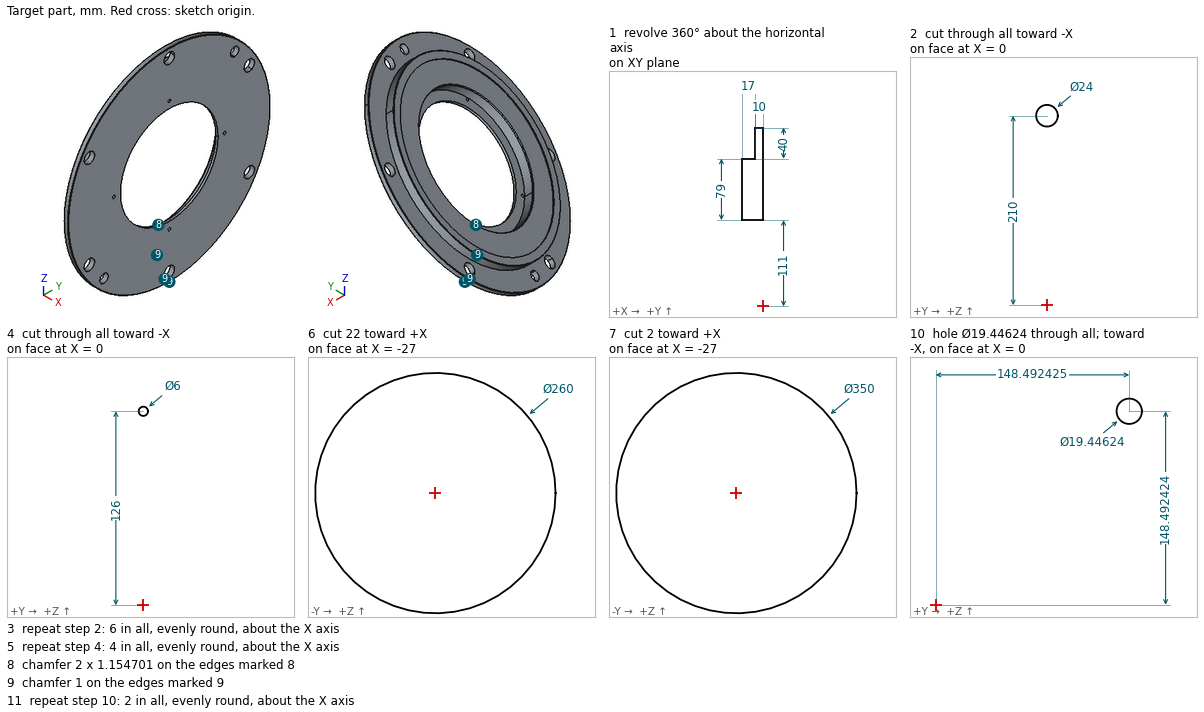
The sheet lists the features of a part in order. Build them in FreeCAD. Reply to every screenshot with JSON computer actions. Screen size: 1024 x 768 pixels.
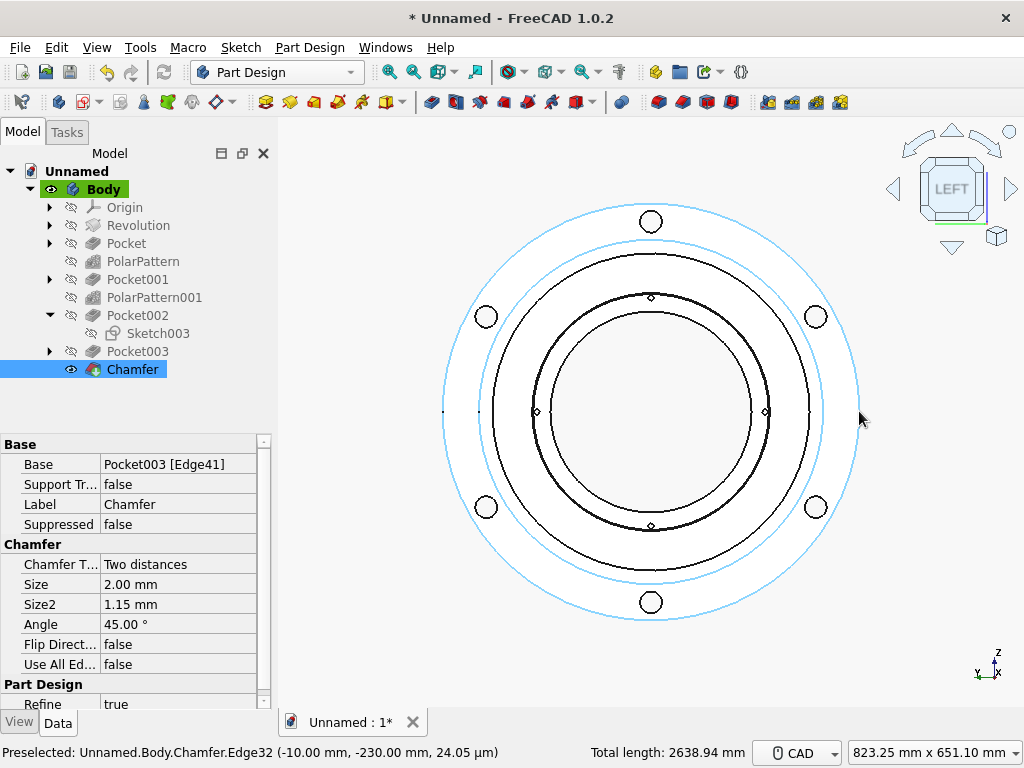
{"action": "key", "text": "0"}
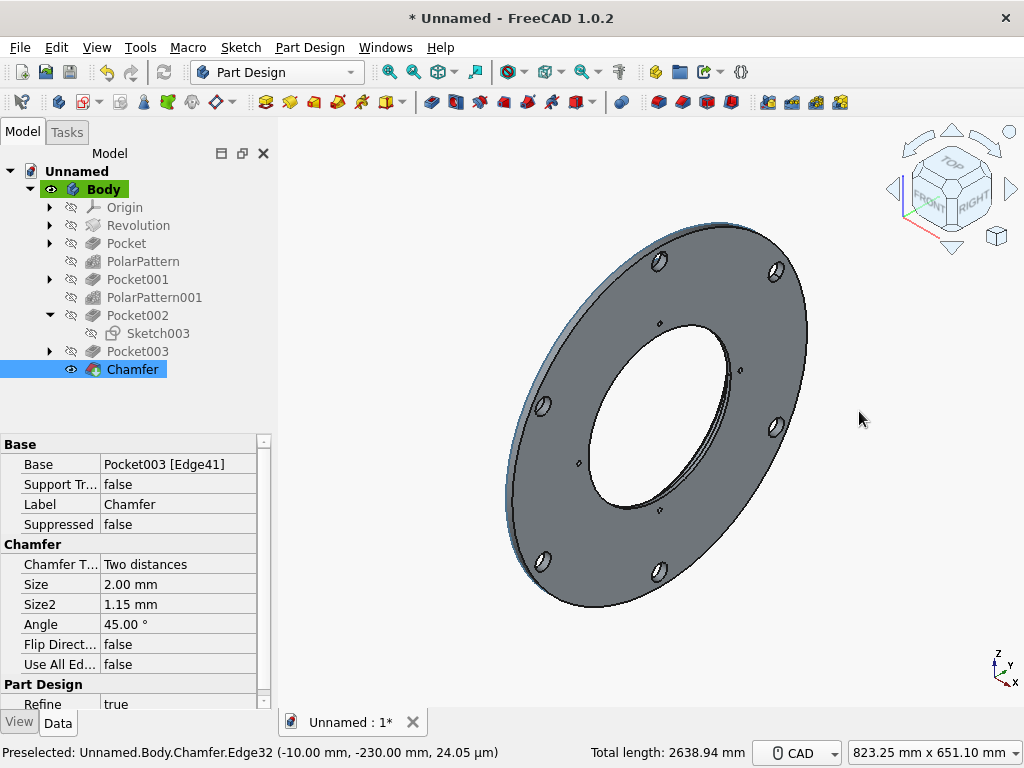
{"action": "left_click", "coordinate": [512, 501], "text": "ctrl"}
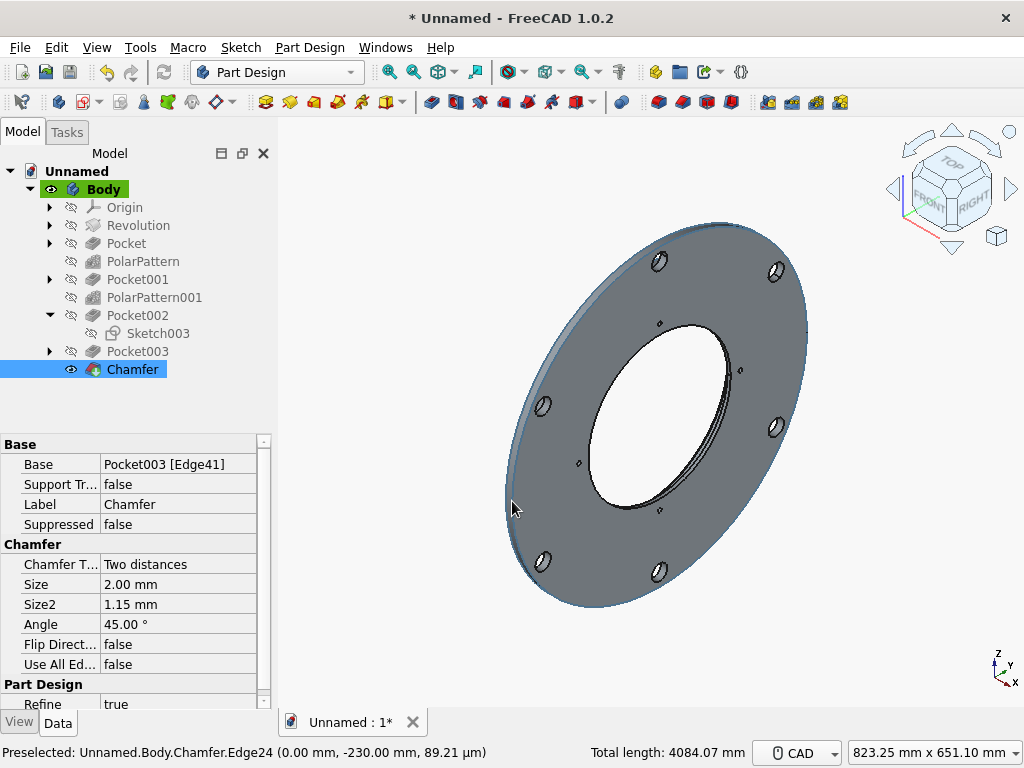
{"action": "left_click", "coordinate": [684, 102]}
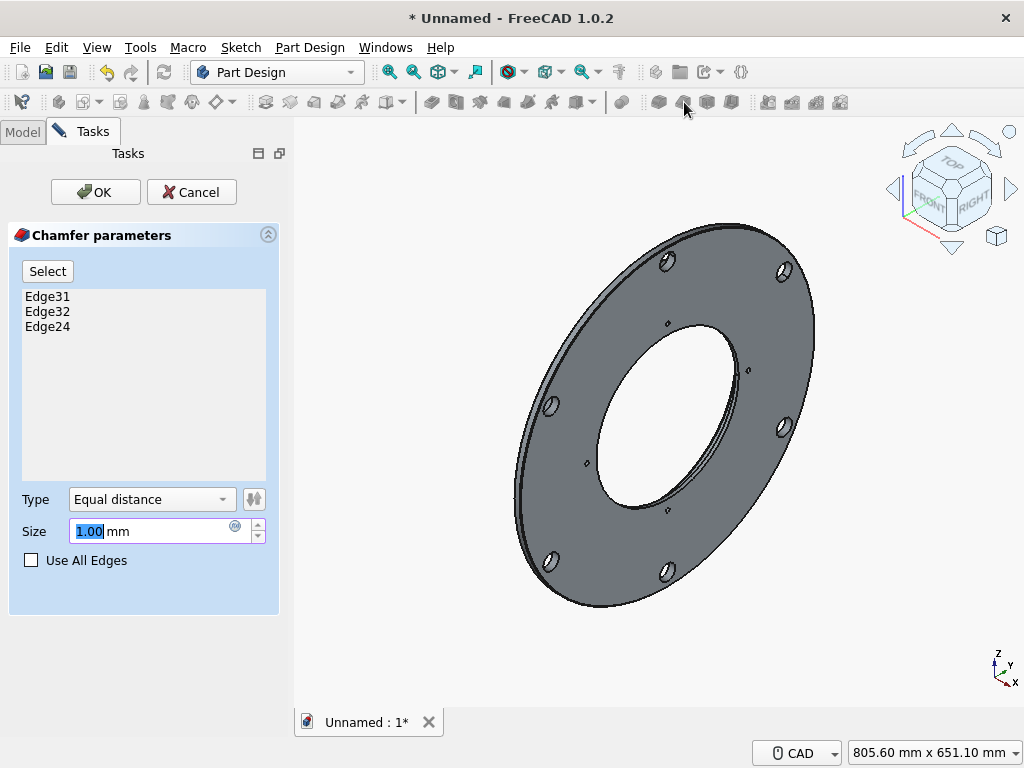
{"action": "type", "text": "1"}
{"action": "key", "text": "Tab"}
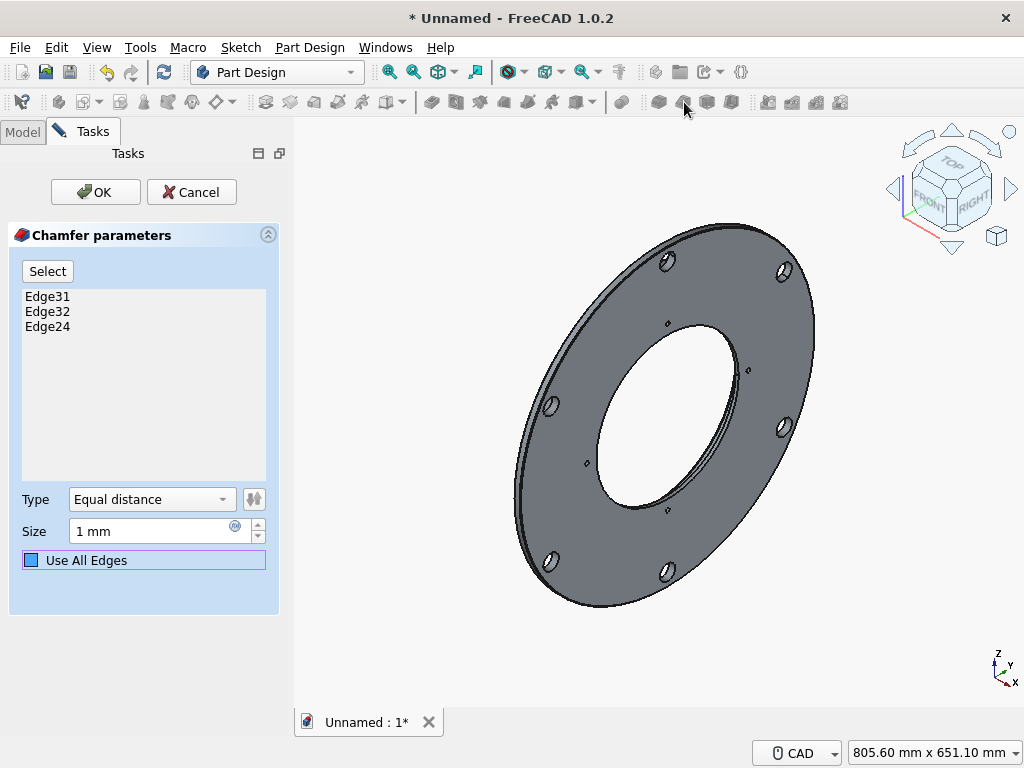
{"action": "left_click", "coordinate": [96, 192]}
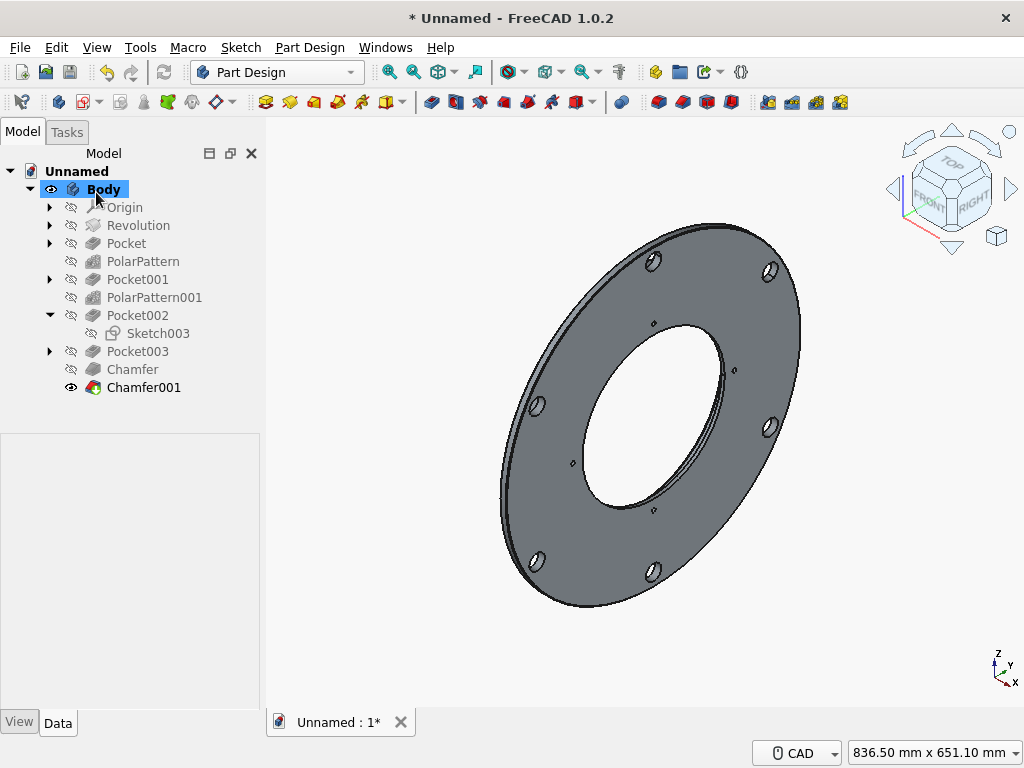
{"action": "left_click", "coordinate": [737, 271]}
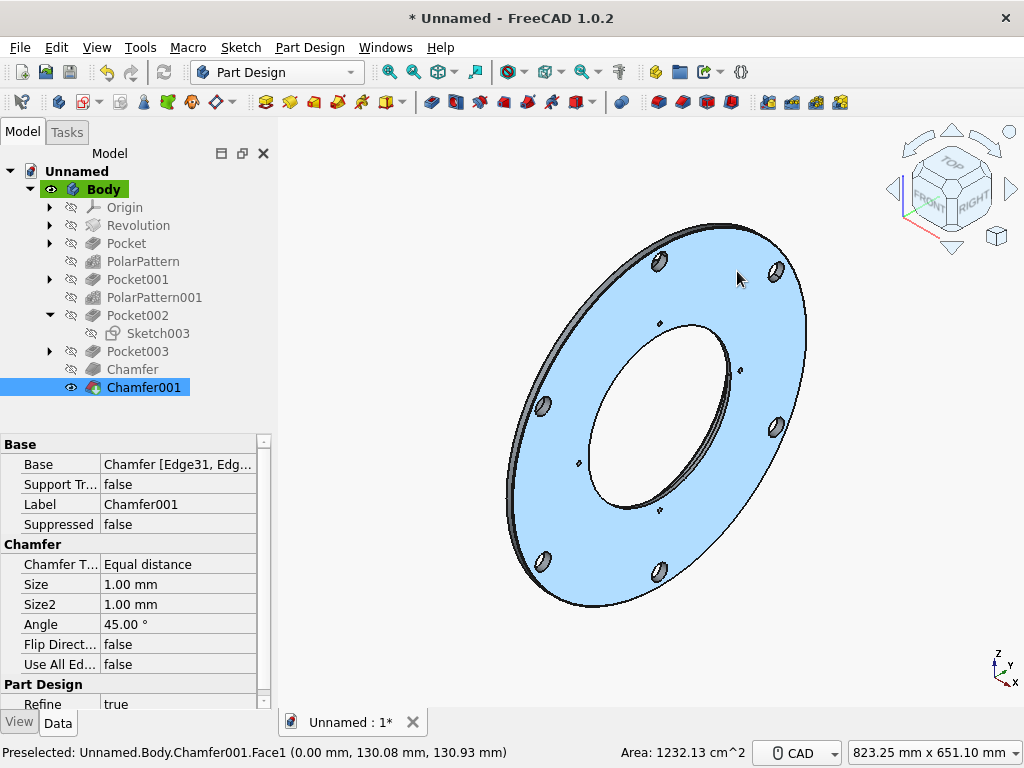
{"action": "left_click", "coordinate": [84, 102]}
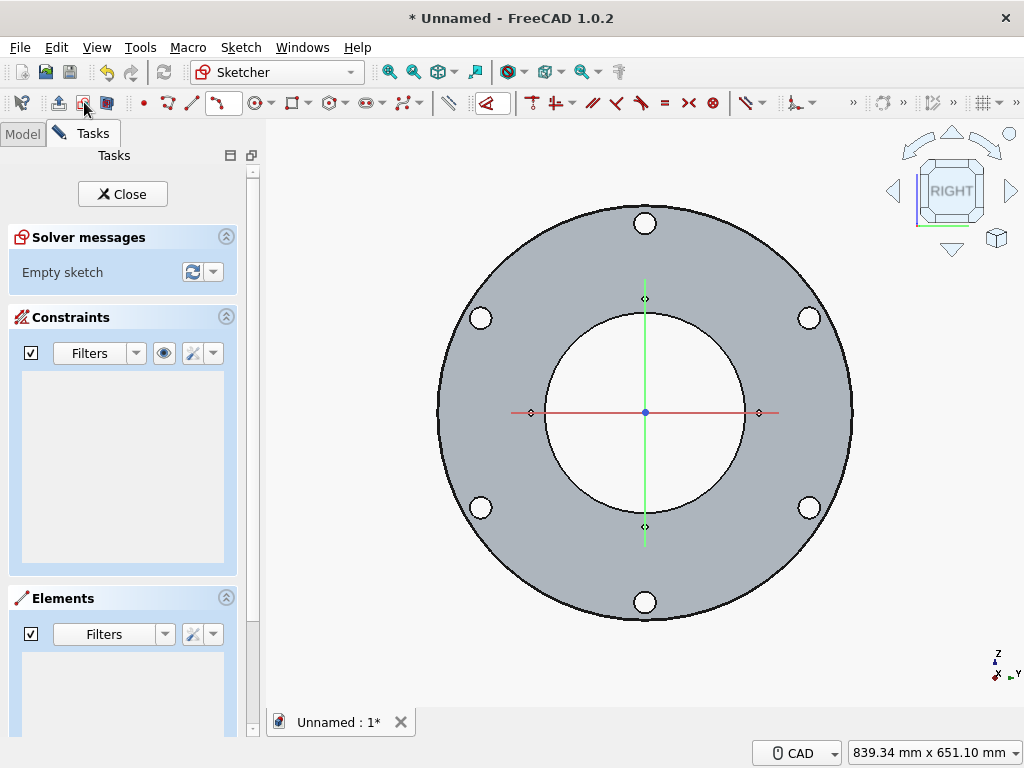
{"action": "scroll", "coordinate": [790, 272], "scroll_direction": "up", "scroll_amount": 15}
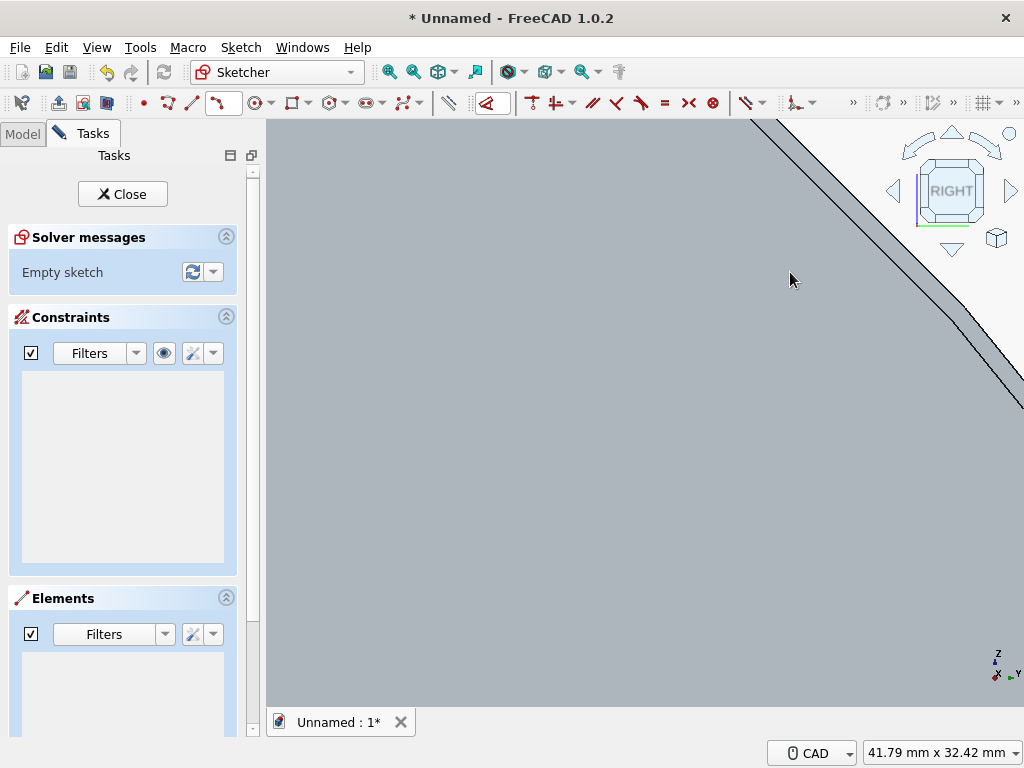
{"action": "left_click", "coordinate": [256, 104]}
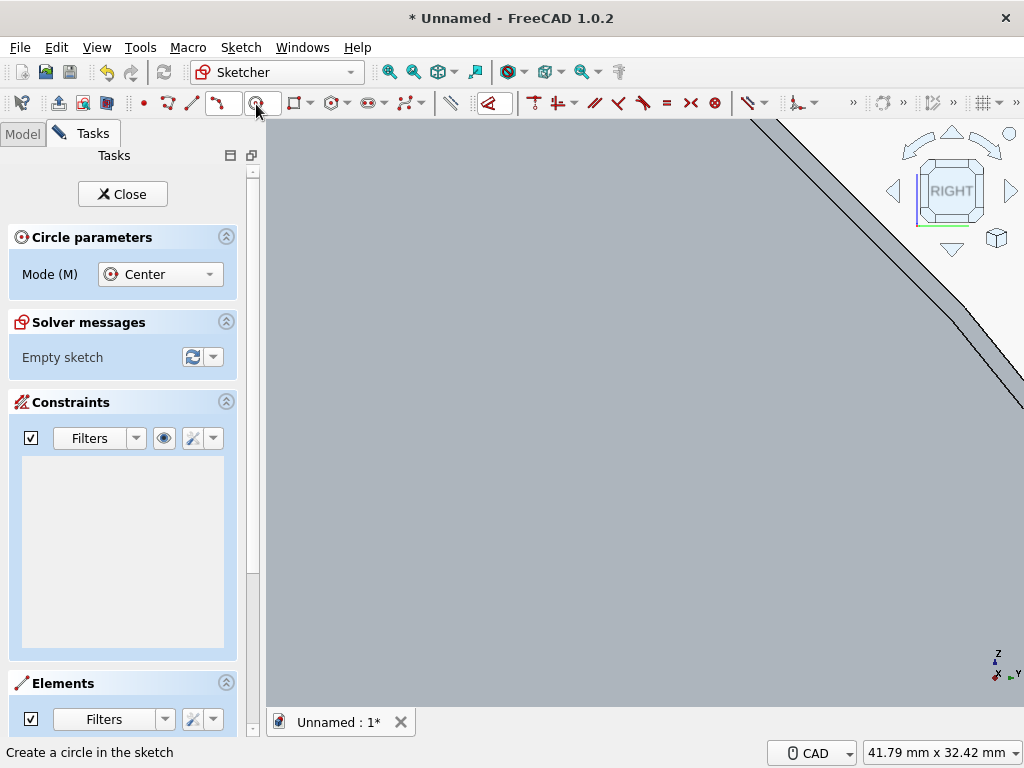
{"action": "left_click", "coordinate": [558, 406]}
{"action": "mouse_move", "coordinate": [683, 281]}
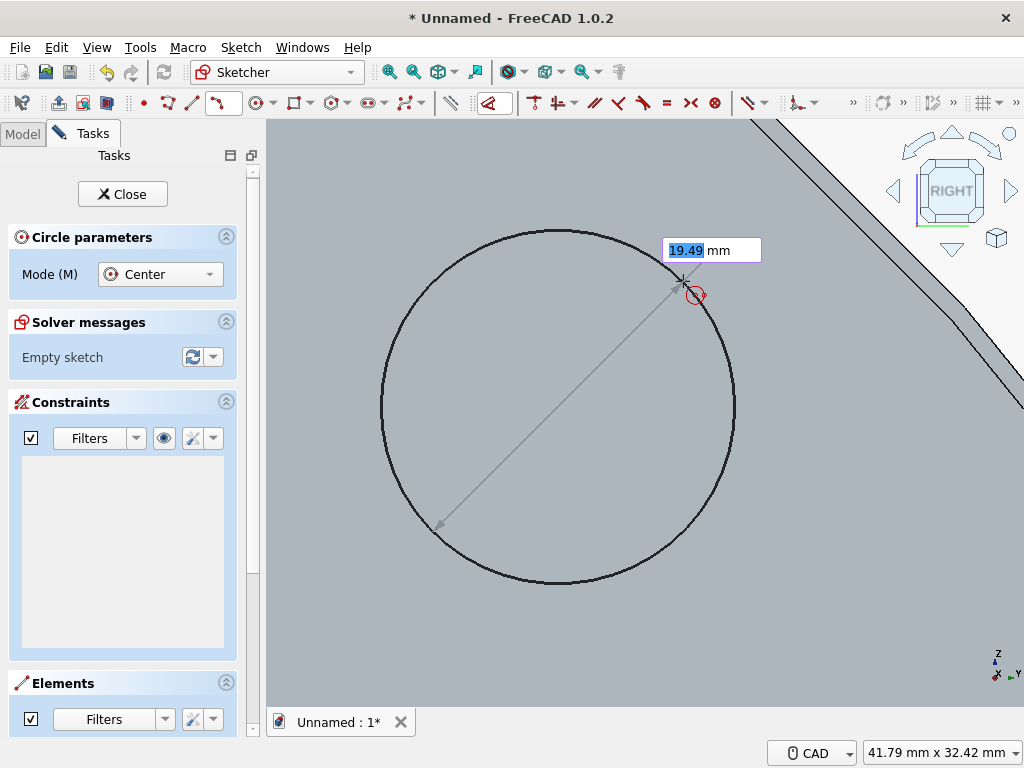
{"action": "type", "text": "19.44624"}
{"action": "key", "text": "Return"}
{"action": "key", "text": "Escape"}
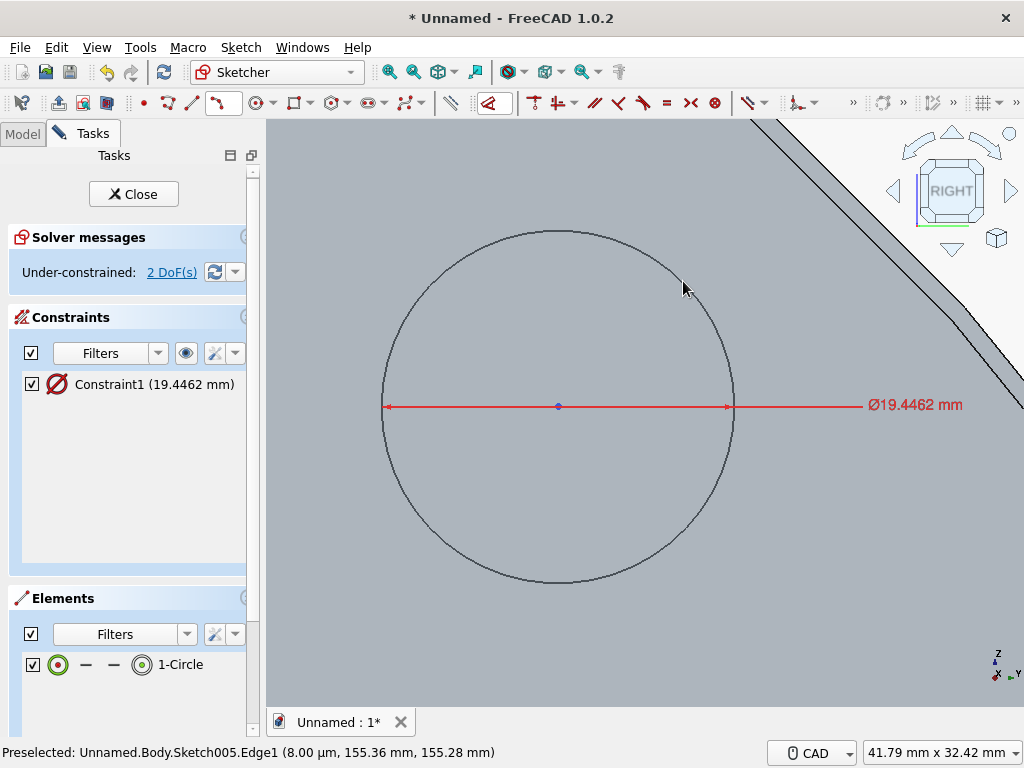
{"action": "key", "text": "d"}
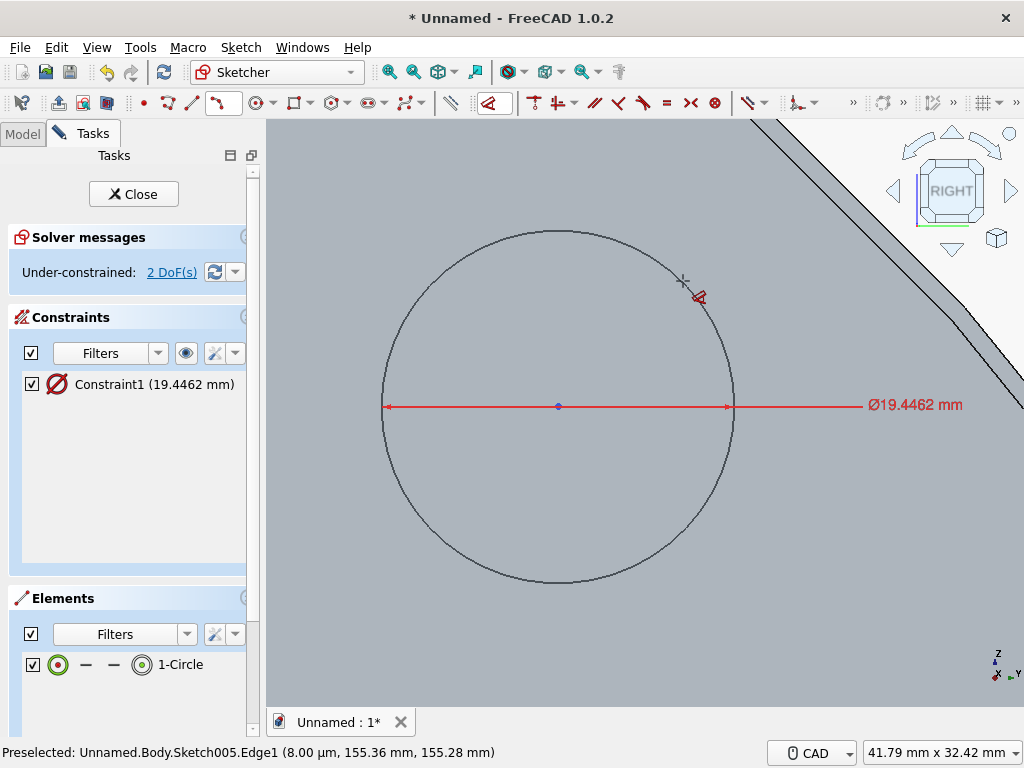
{"action": "left_click", "coordinate": [558, 407]}
{"action": "left_click", "coordinate": [426, 373]}